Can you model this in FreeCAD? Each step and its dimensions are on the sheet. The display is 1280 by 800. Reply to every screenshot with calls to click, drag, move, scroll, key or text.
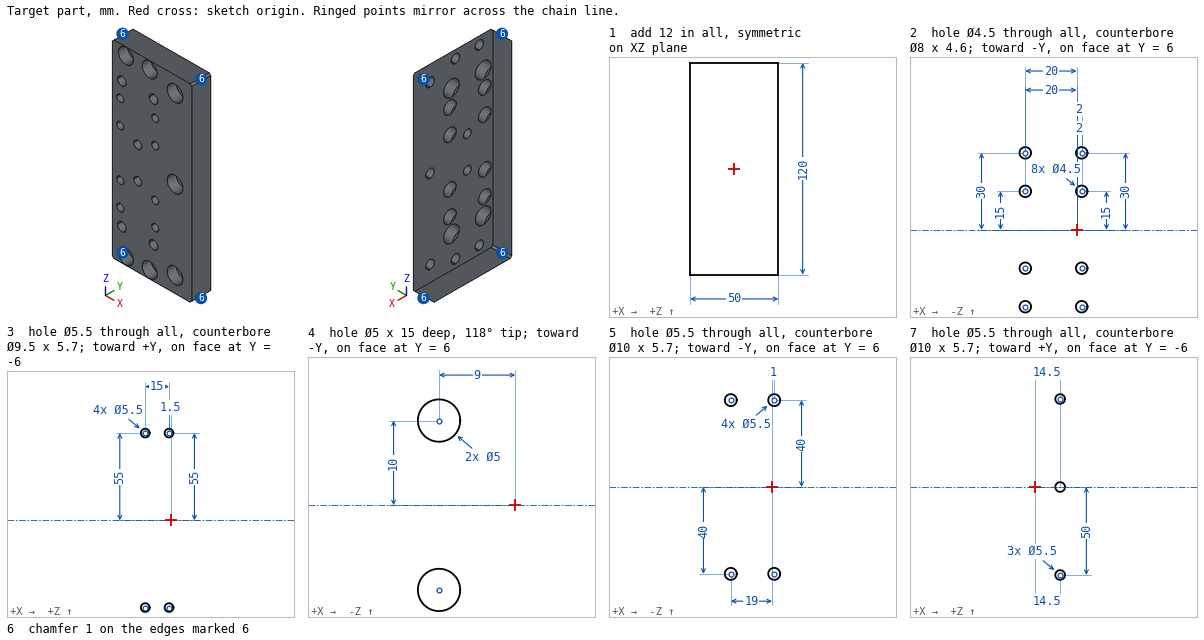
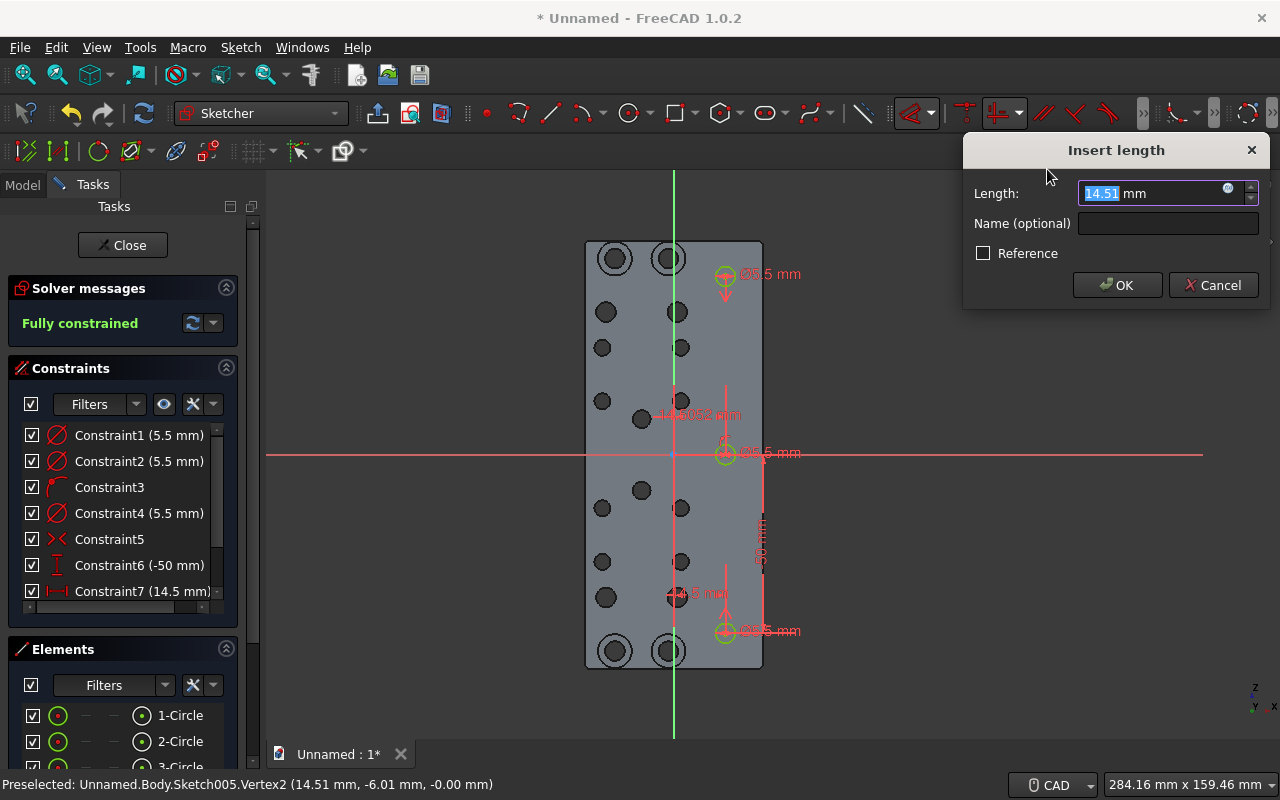
text(14.5)
key(Return)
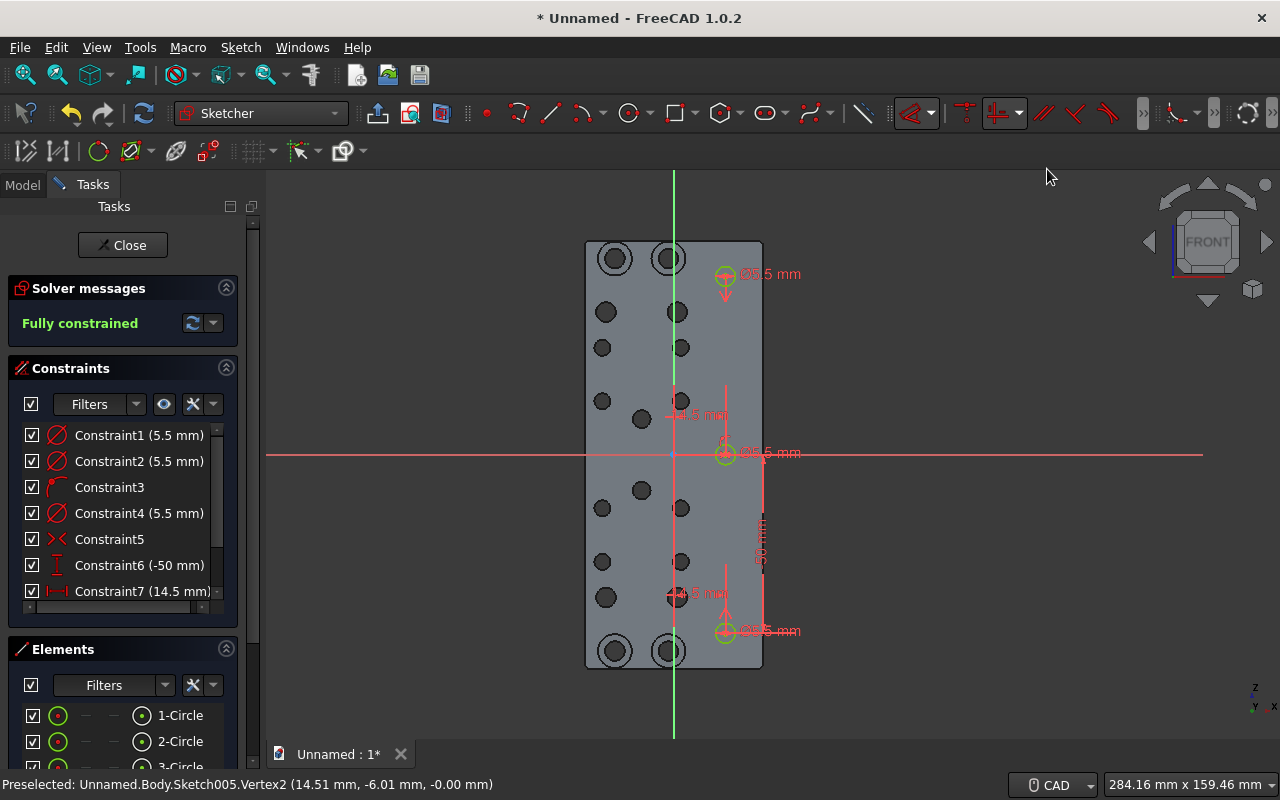
click(123, 245)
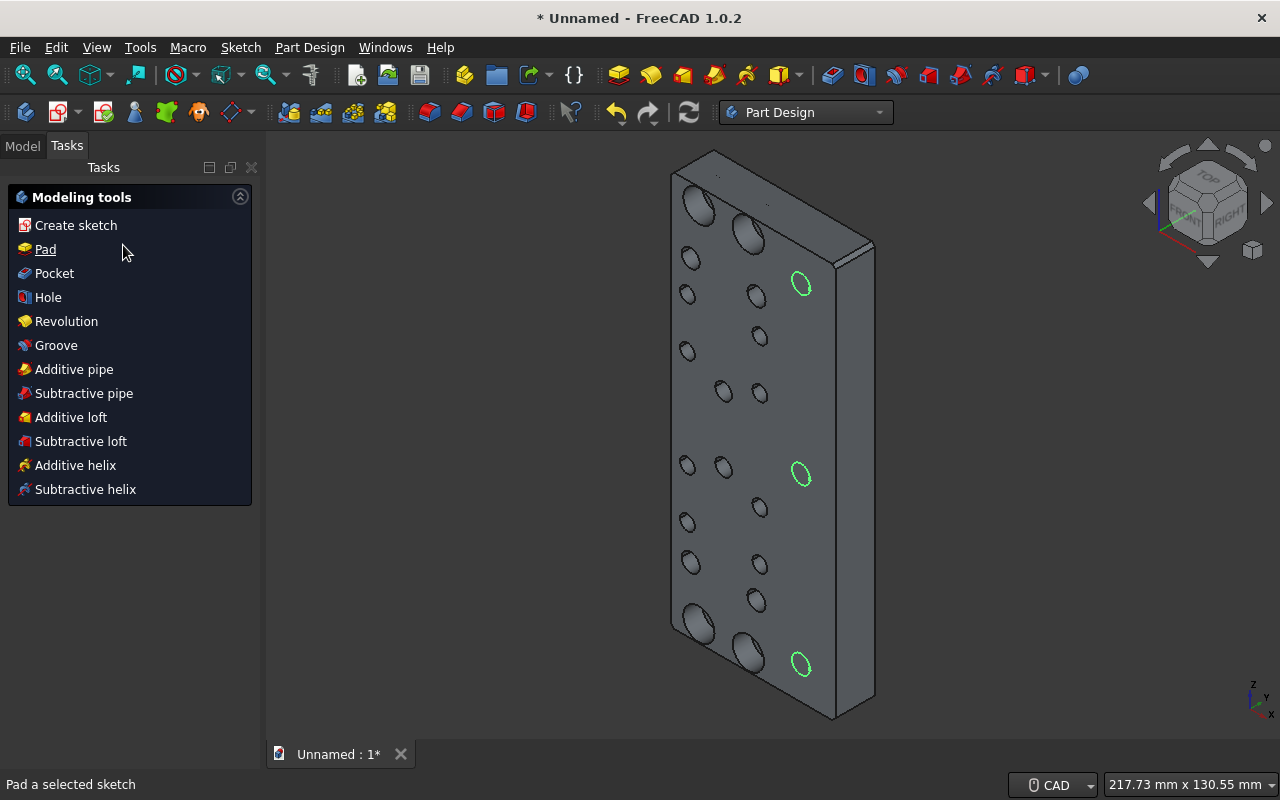
click(866, 76)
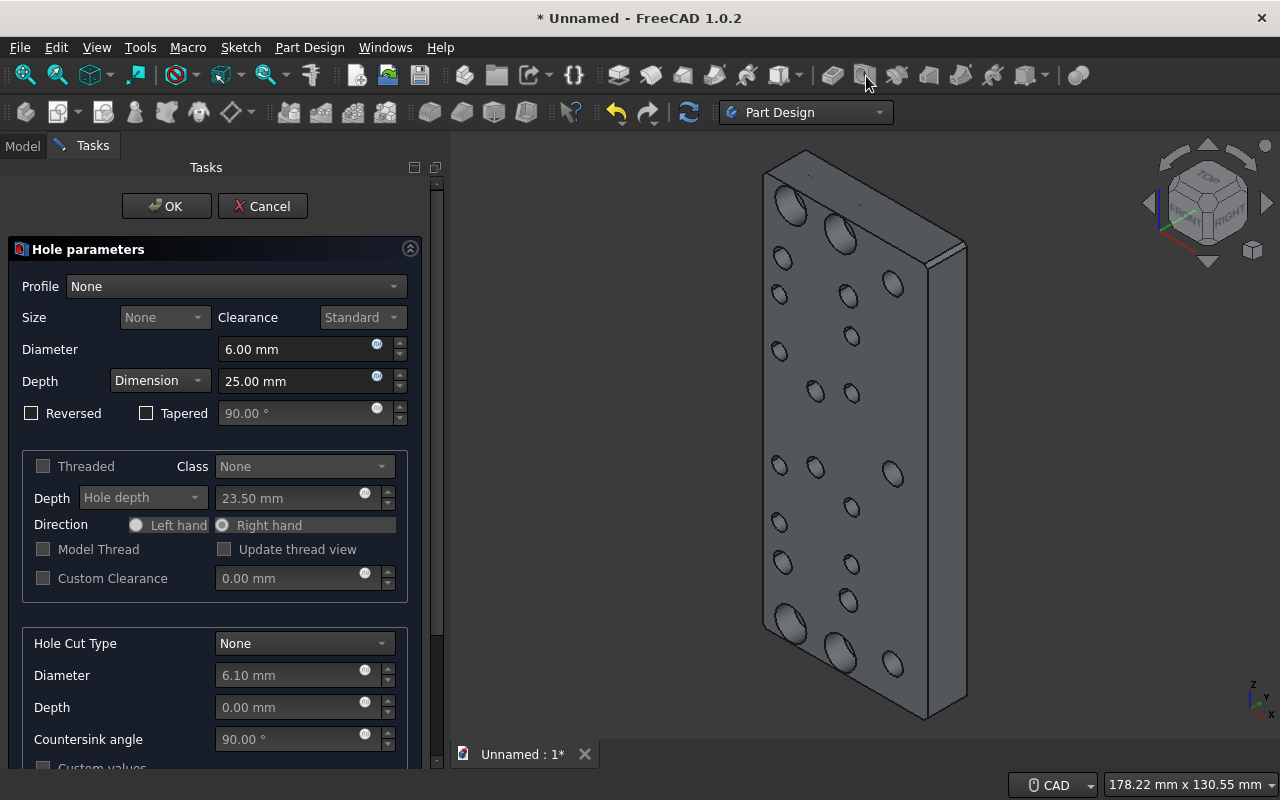
triple_click(305, 349)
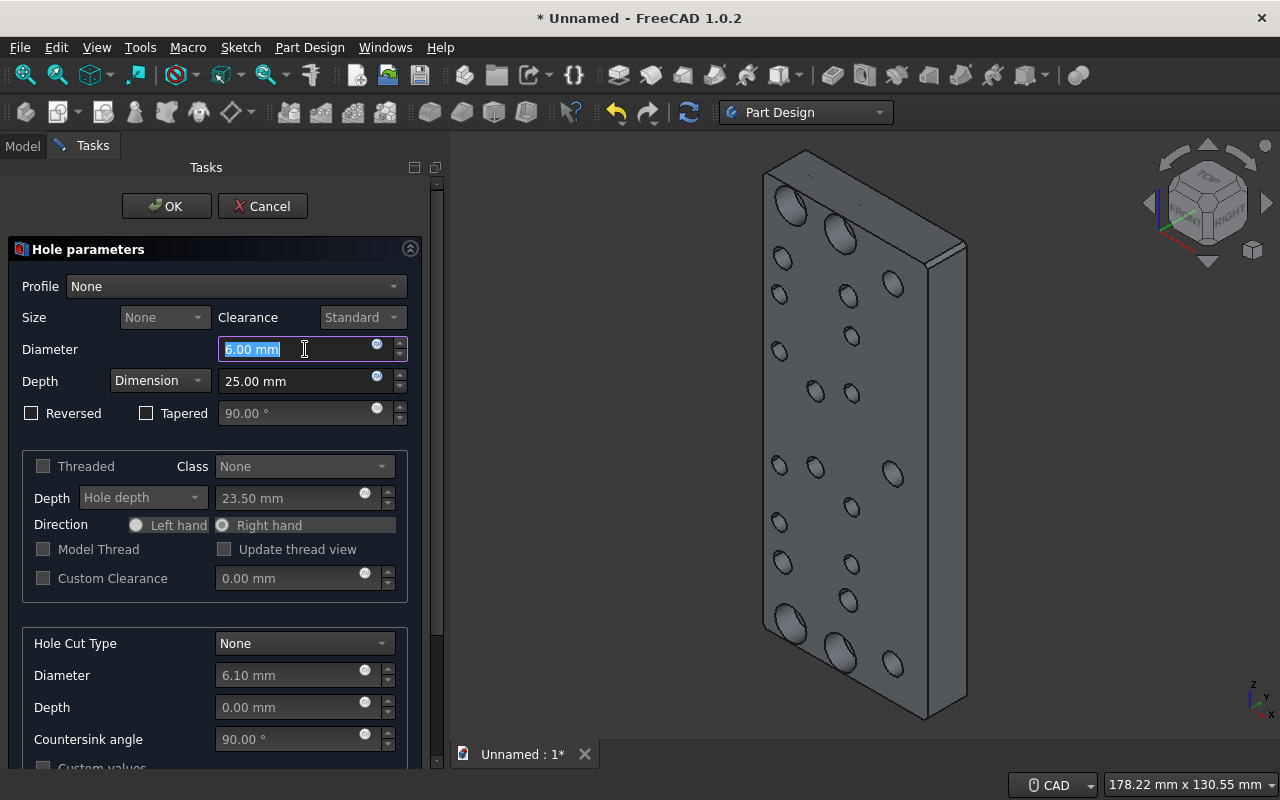
text(5.5)
key(Tab)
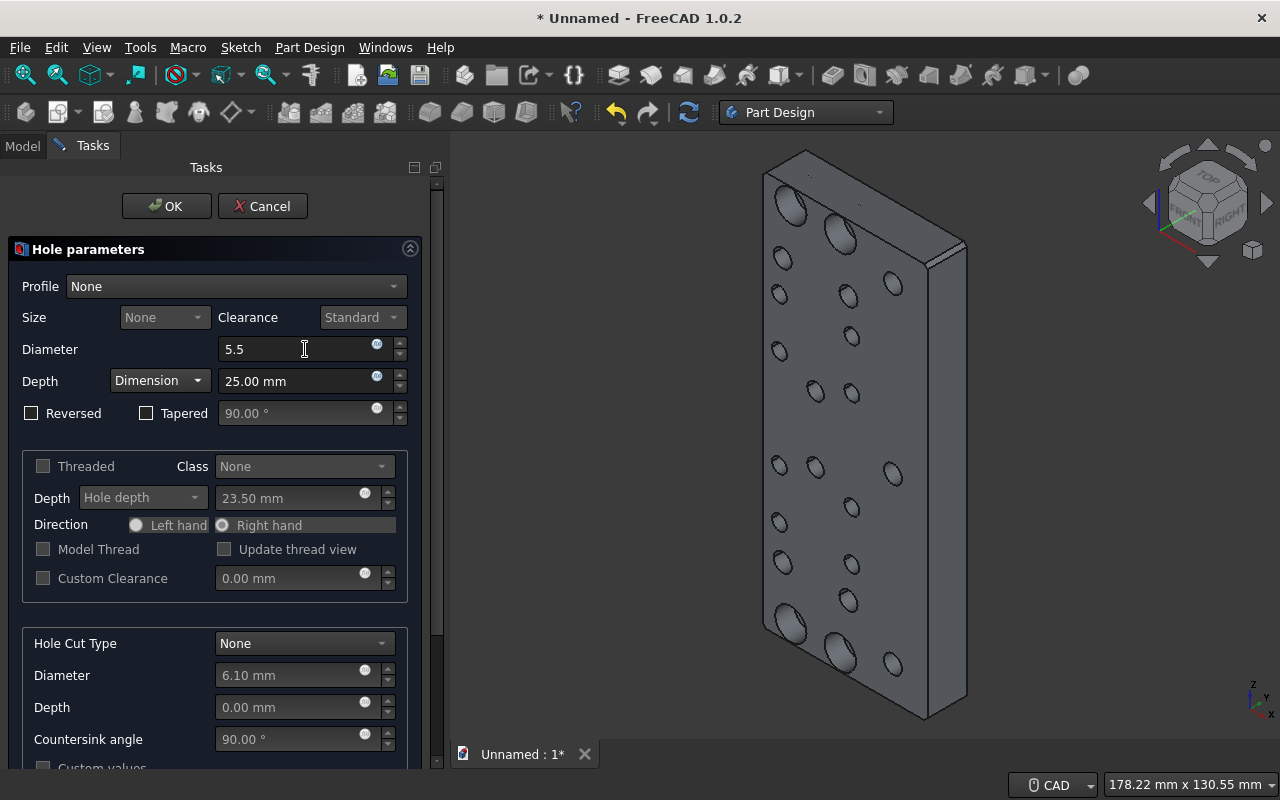
click(161, 380)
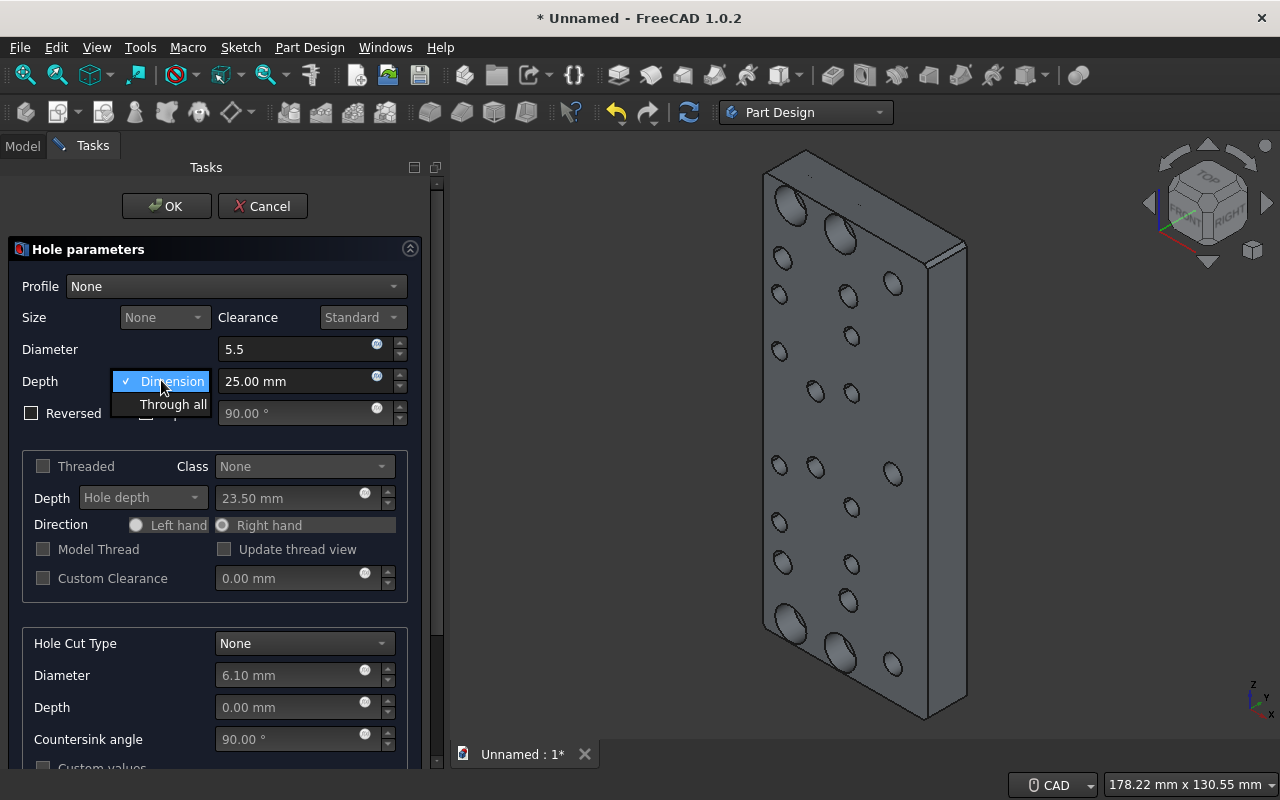
click(160, 404)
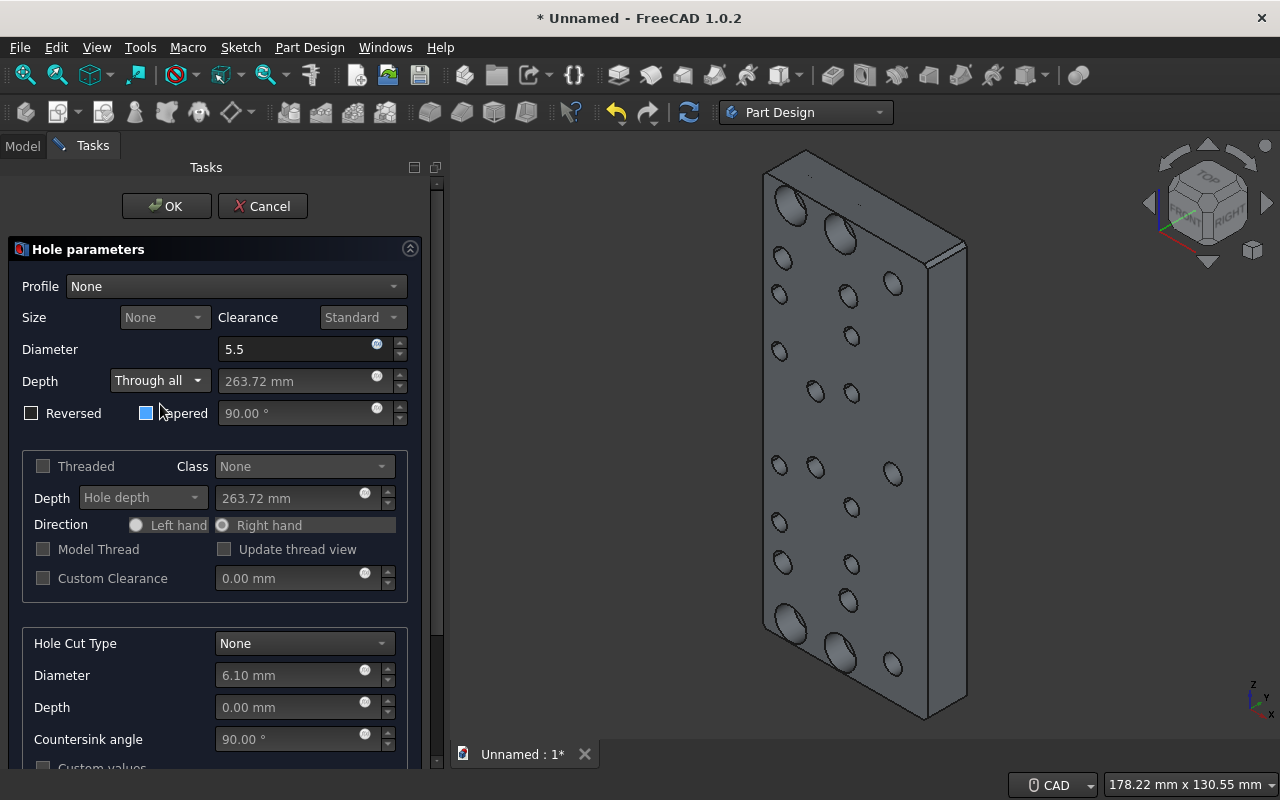
click(306, 644)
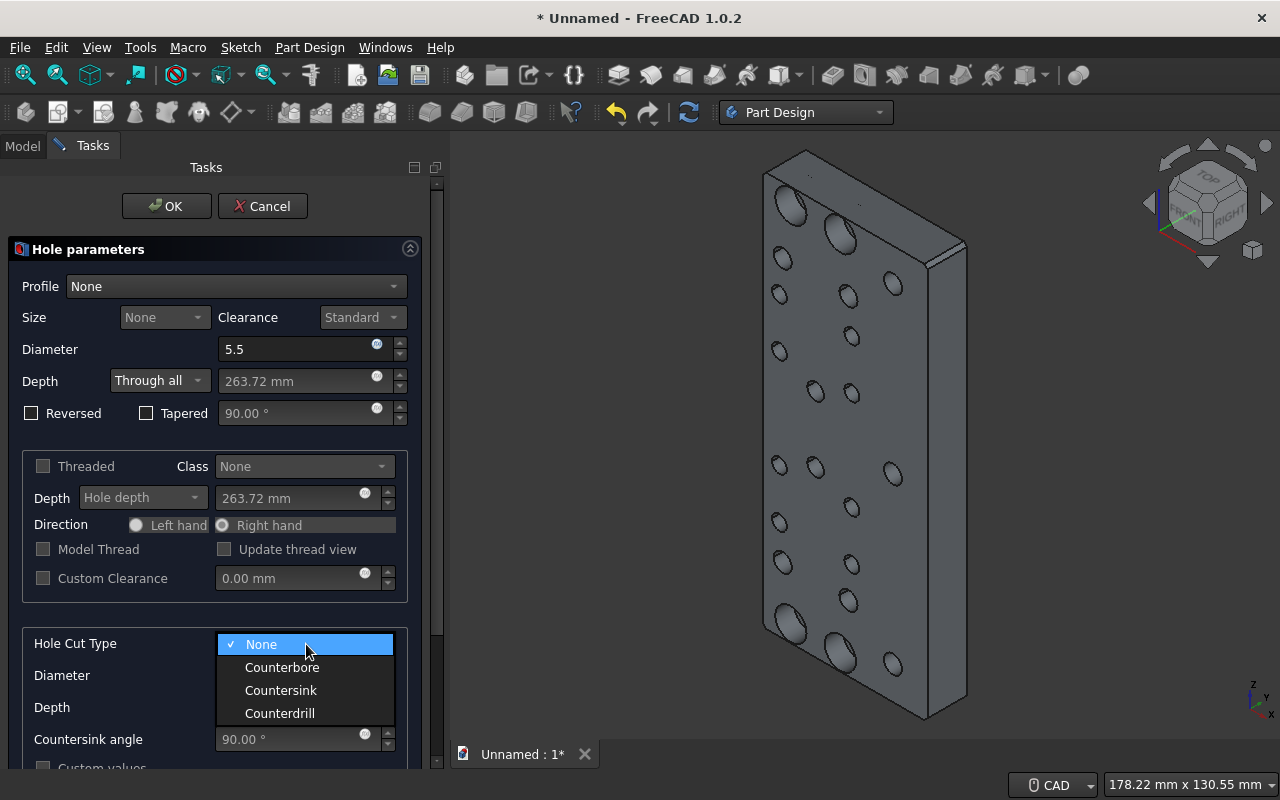
click(304, 668)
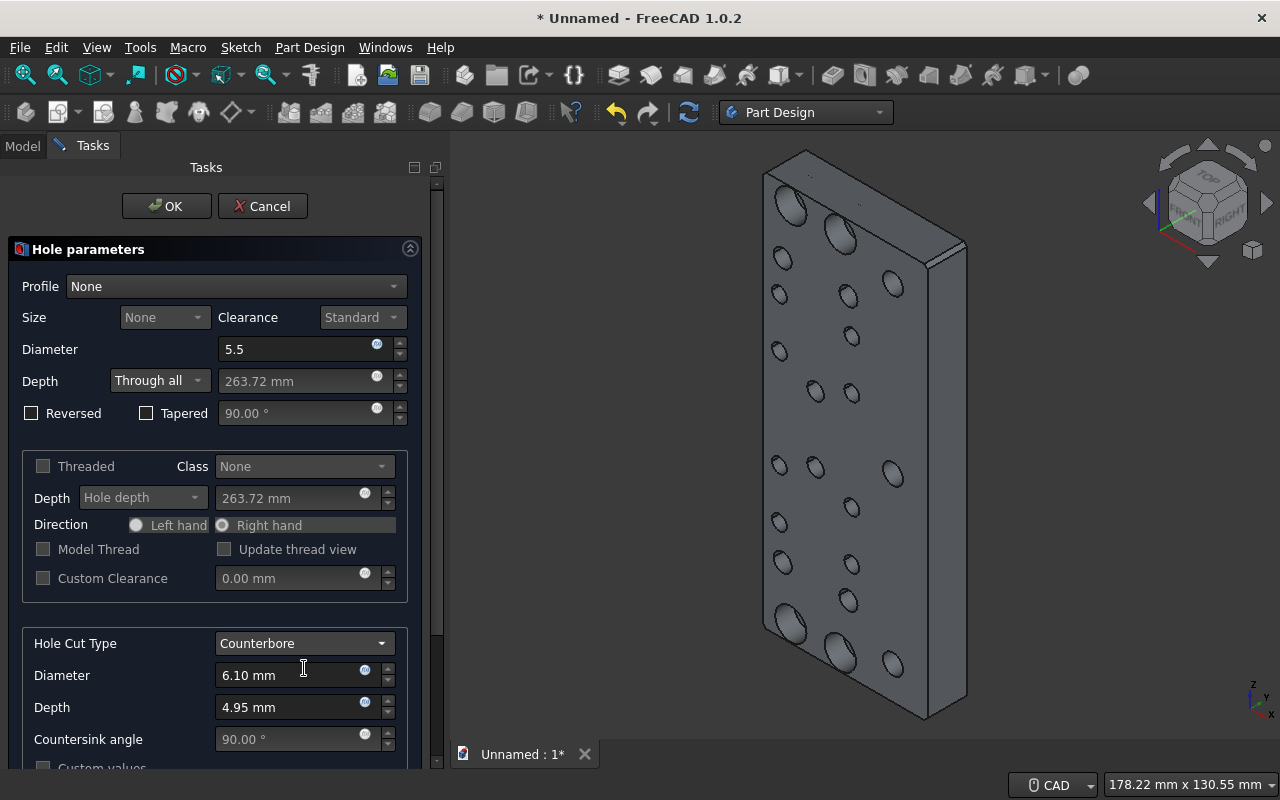
triple_click(298, 675)